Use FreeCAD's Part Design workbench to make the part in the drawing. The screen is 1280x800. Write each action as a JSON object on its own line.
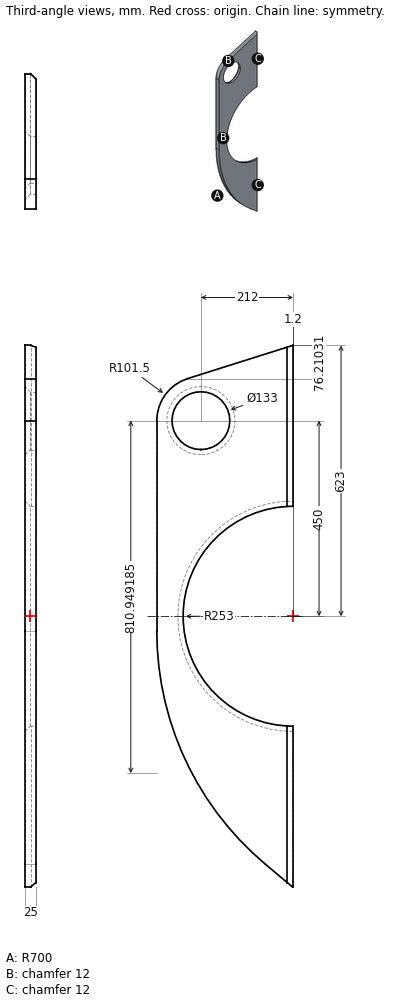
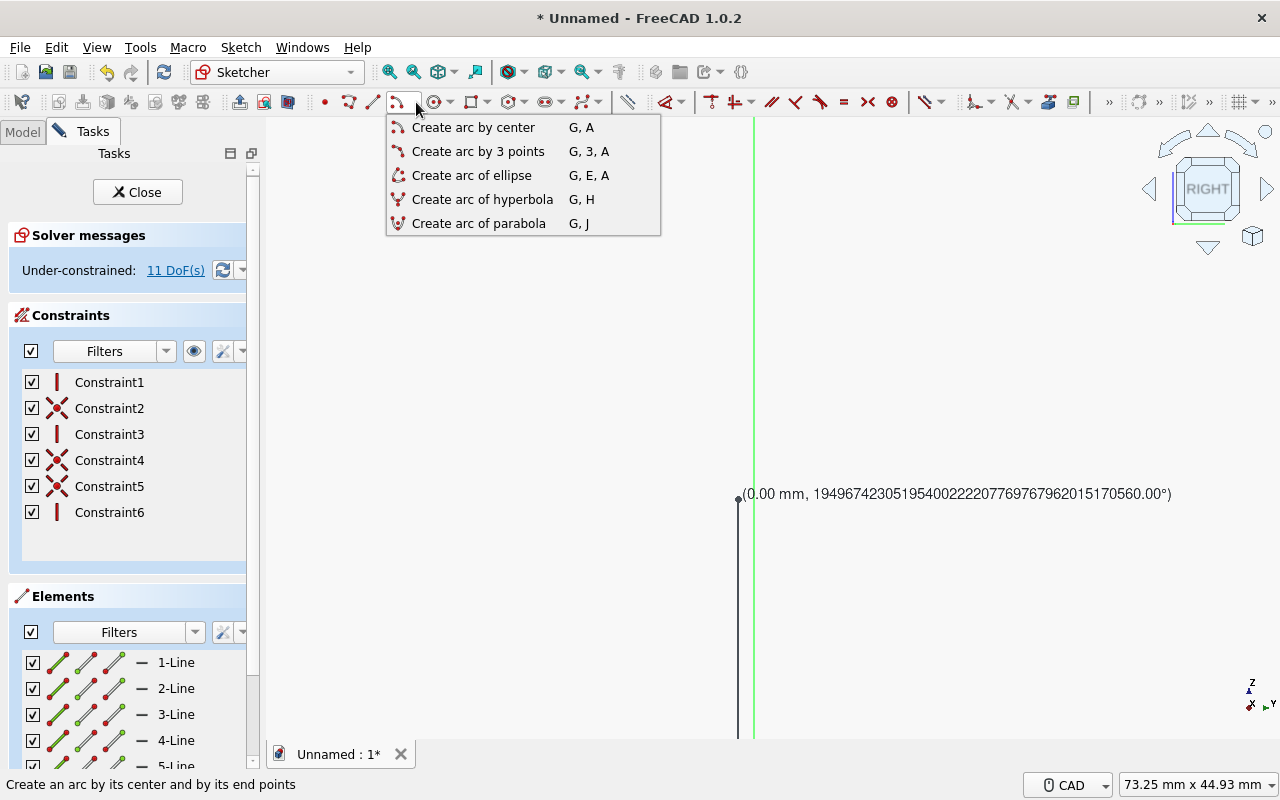
{"action": "left_click", "coordinate": [524, 151]}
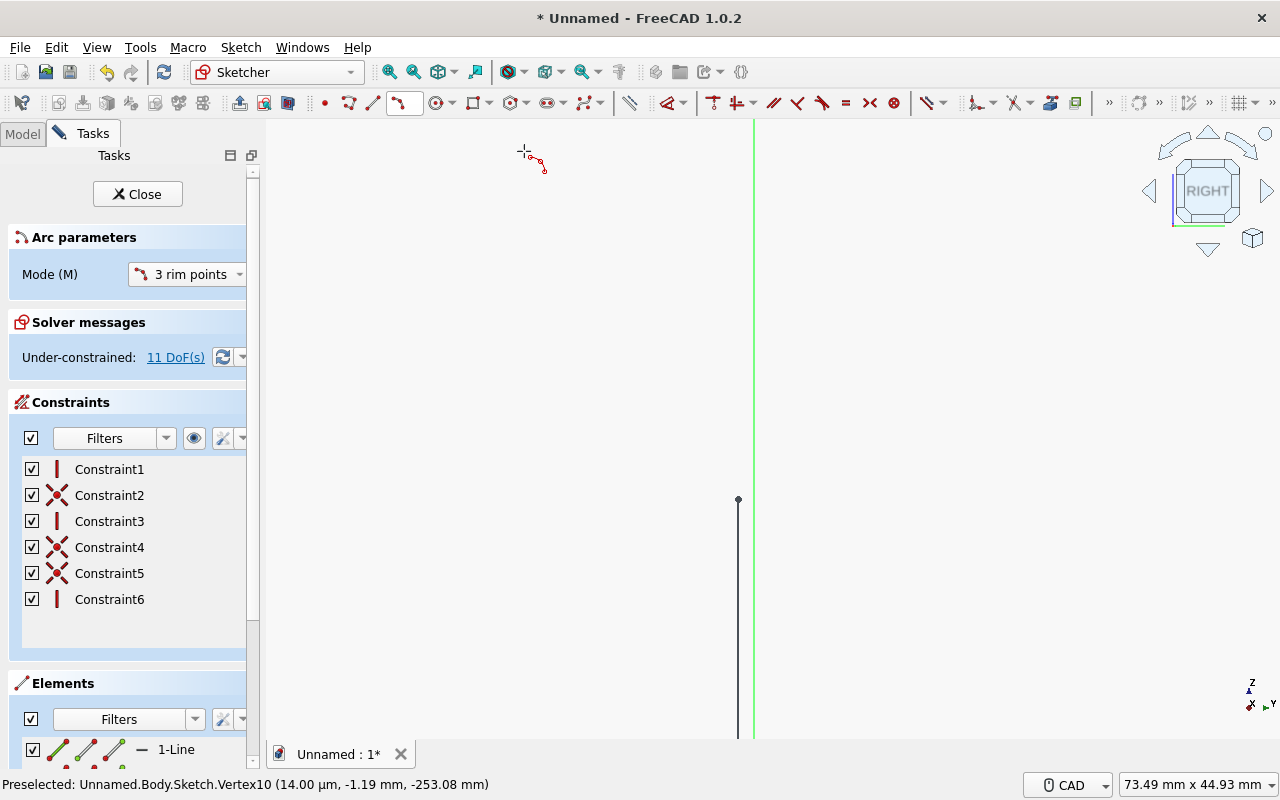
{"action": "scroll", "coordinate": [764, 525], "scroll_direction": "down", "scroll_amount": 18}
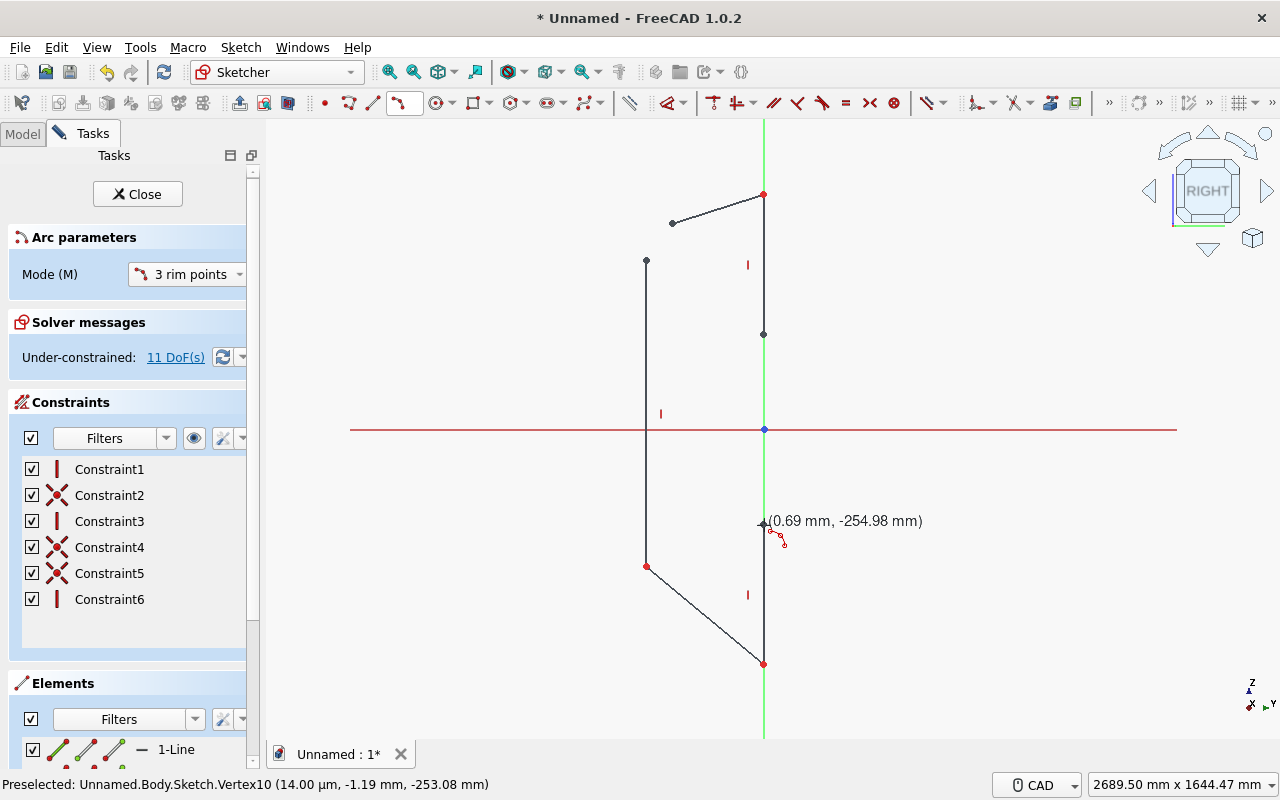
{"action": "left_click", "coordinate": [672, 224]}
{"action": "left_click", "coordinate": [646, 261]}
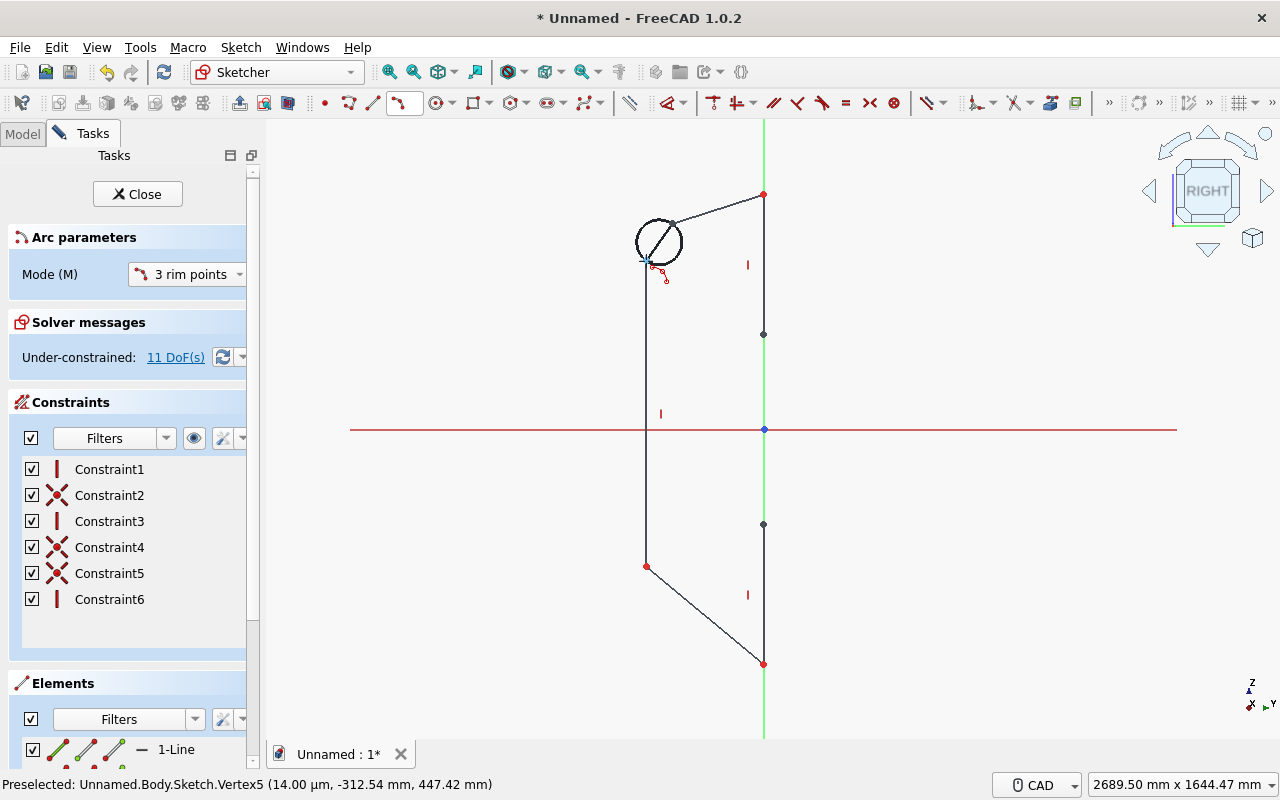
{"action": "scroll", "coordinate": [653, 237], "scroll_direction": "up", "scroll_amount": 4}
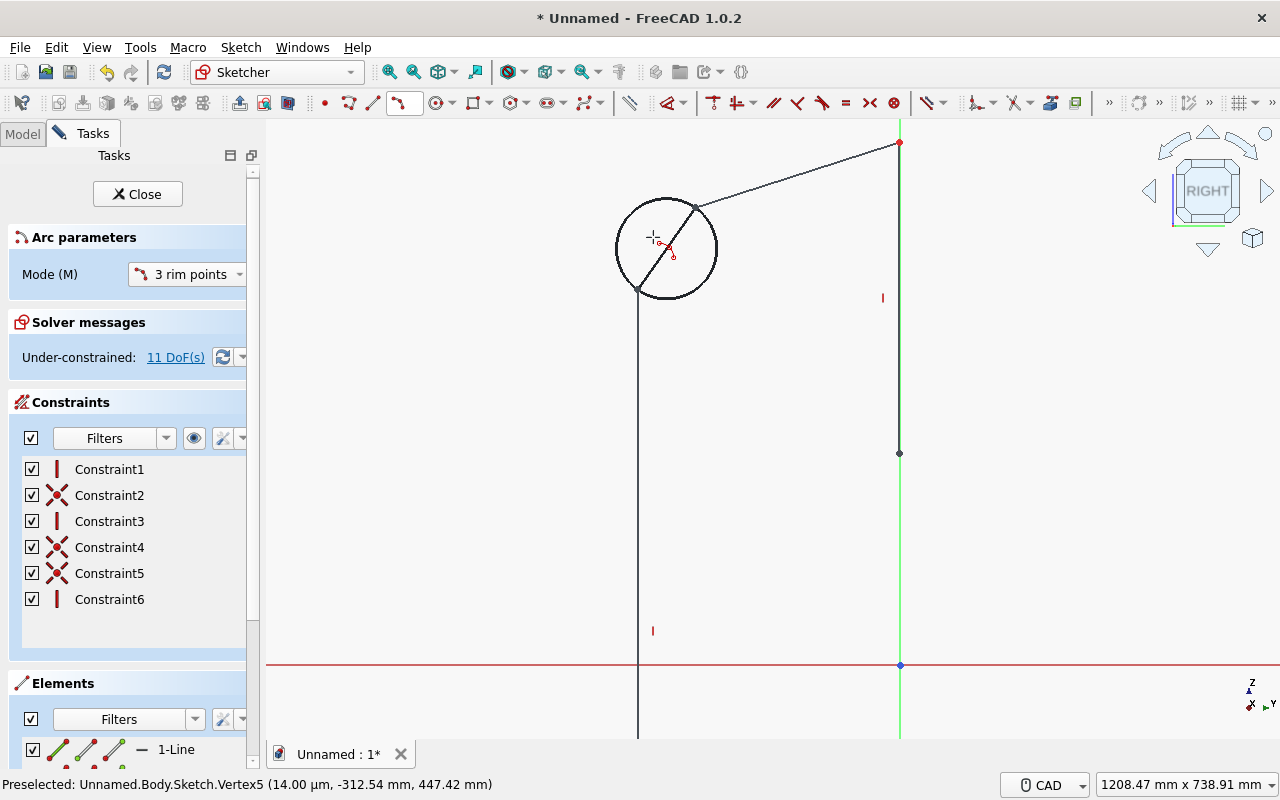
{"action": "left_click", "coordinate": [653, 237]}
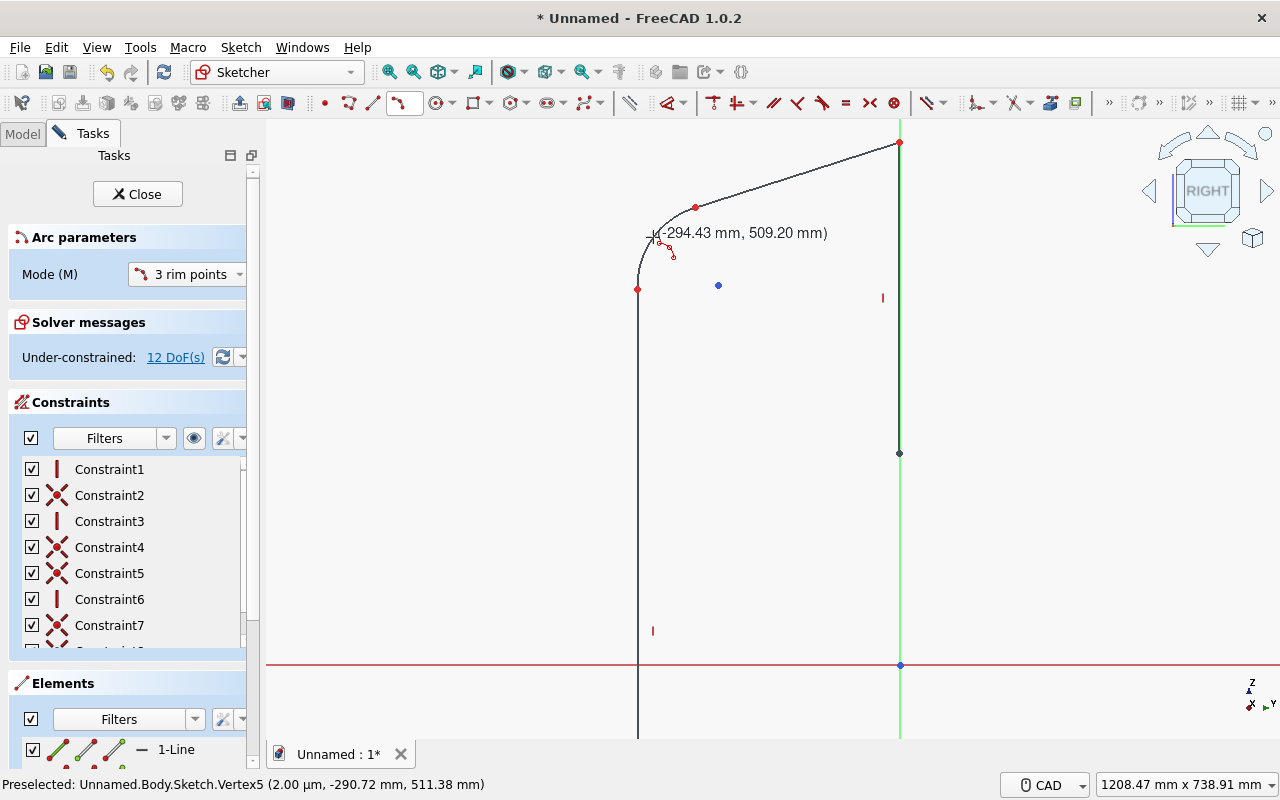
{"action": "scroll", "coordinate": [667, 292], "scroll_direction": "down", "scroll_amount": 5}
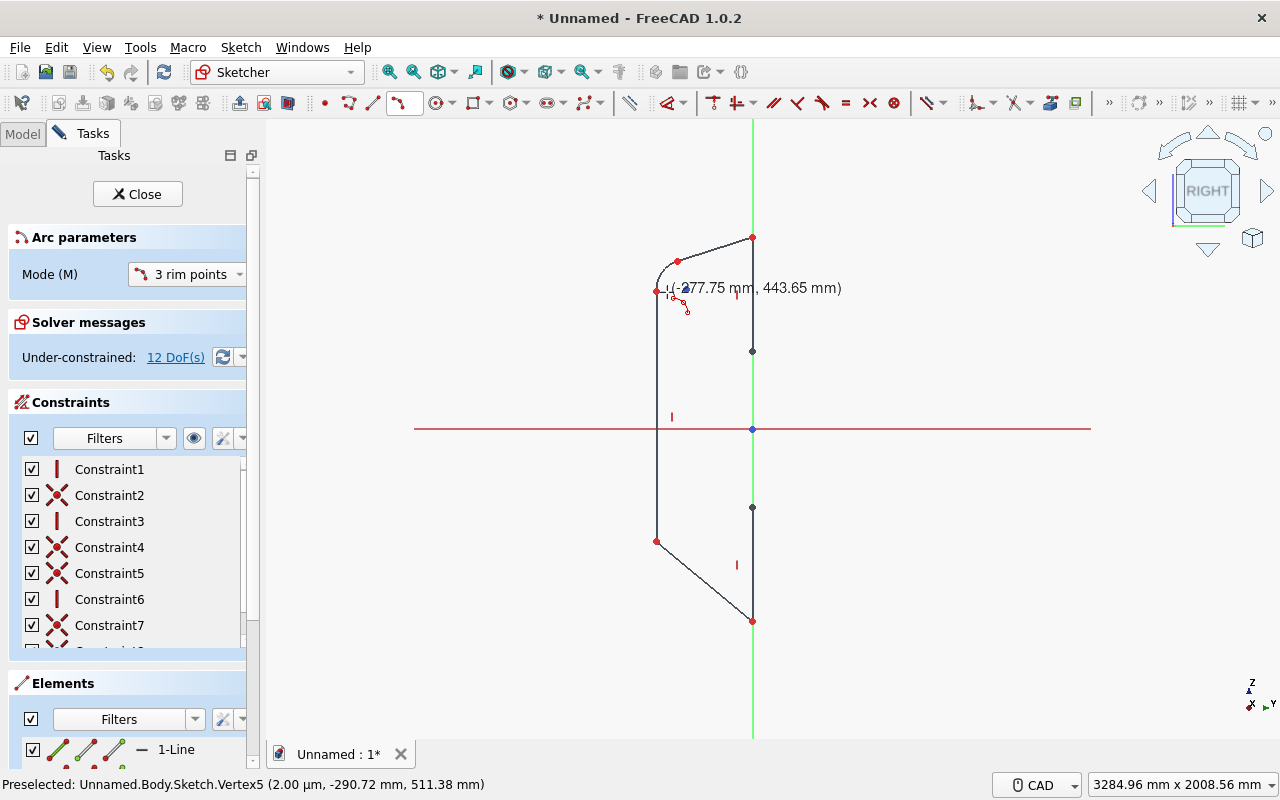
{"action": "scroll", "coordinate": [753, 508], "scroll_direction": "up", "scroll_amount": 19}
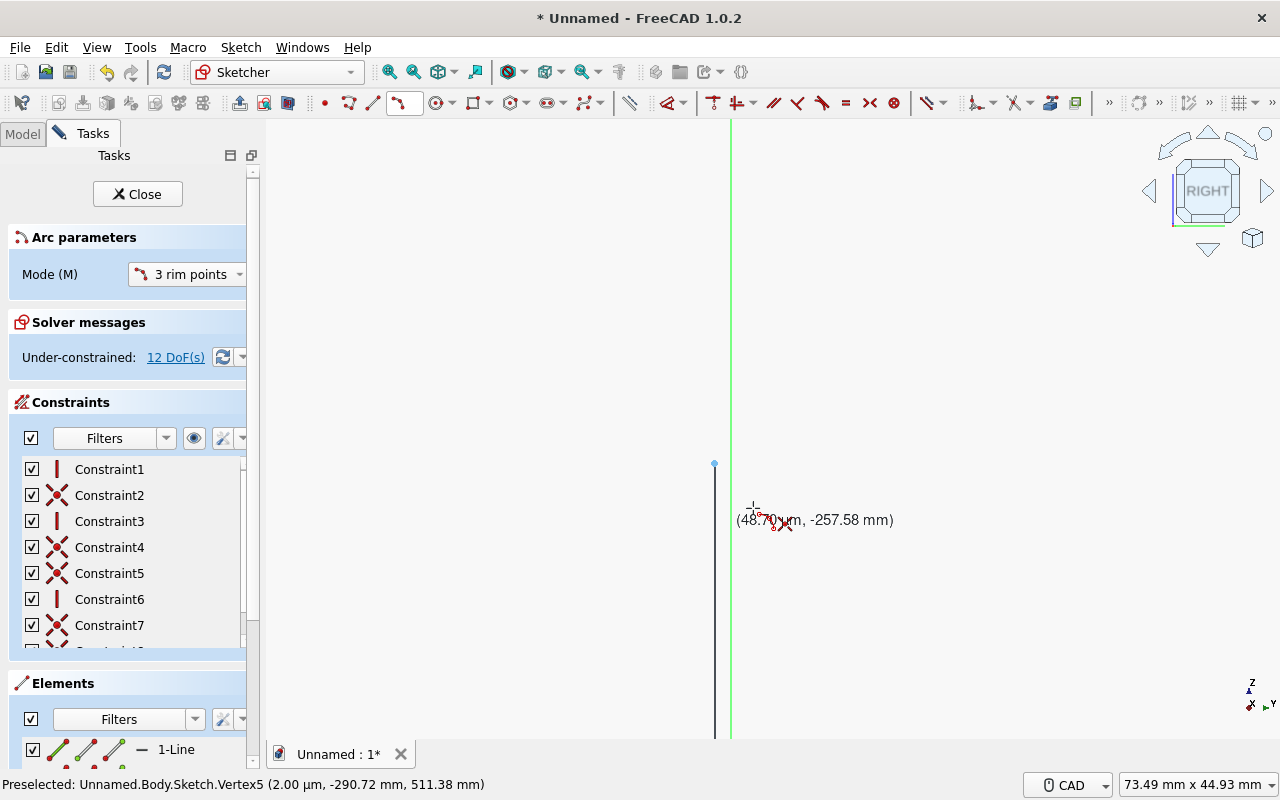
{"action": "left_click", "coordinate": [715, 463]}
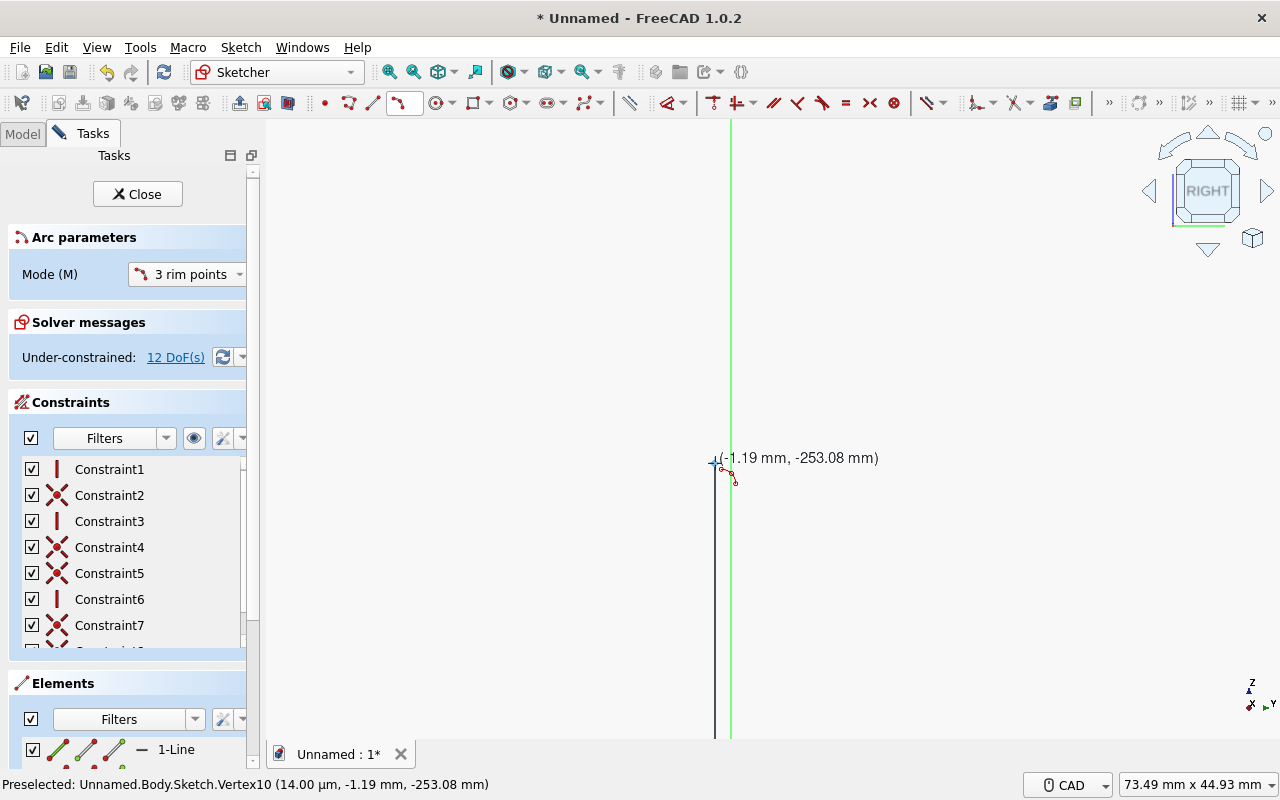
{"action": "scroll", "coordinate": [765, 526], "scroll_direction": "down", "scroll_amount": 18}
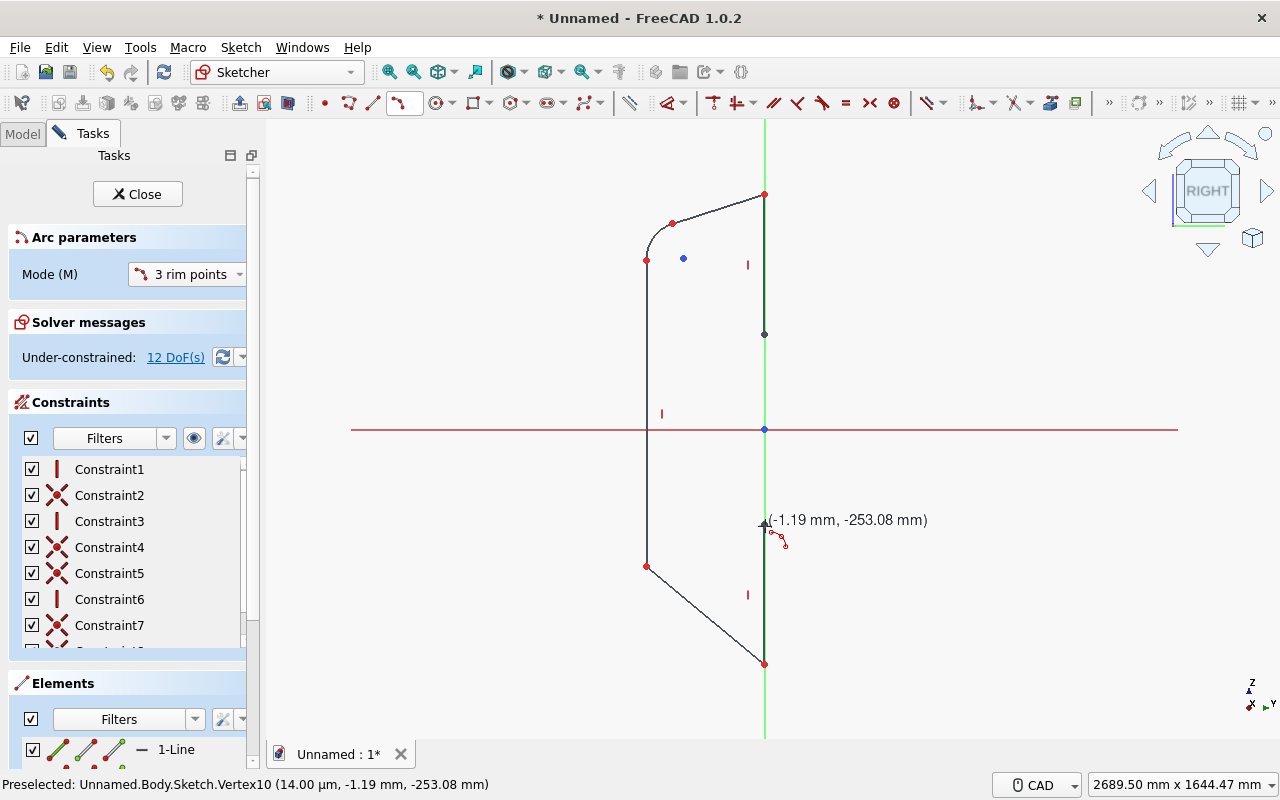
{"action": "scroll", "coordinate": [764, 334], "scroll_direction": "up", "scroll_amount": 18}